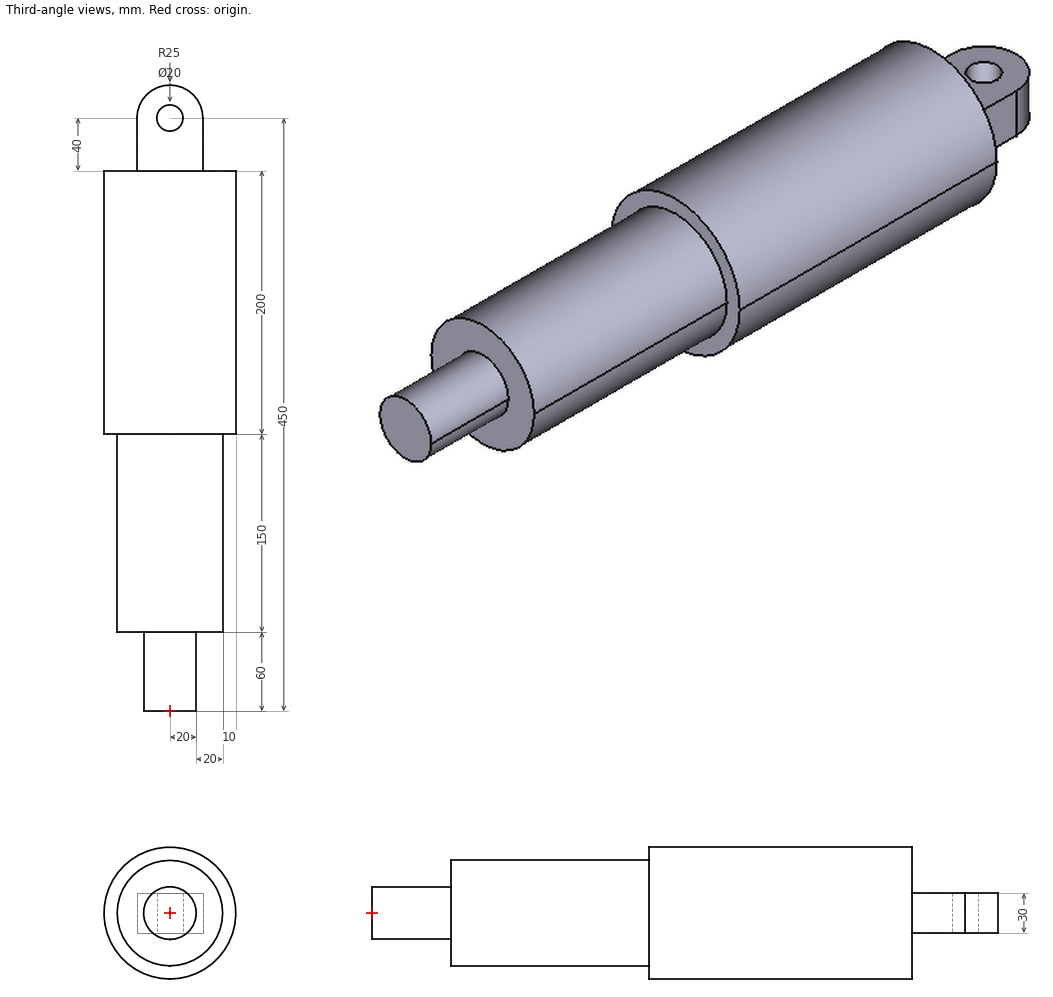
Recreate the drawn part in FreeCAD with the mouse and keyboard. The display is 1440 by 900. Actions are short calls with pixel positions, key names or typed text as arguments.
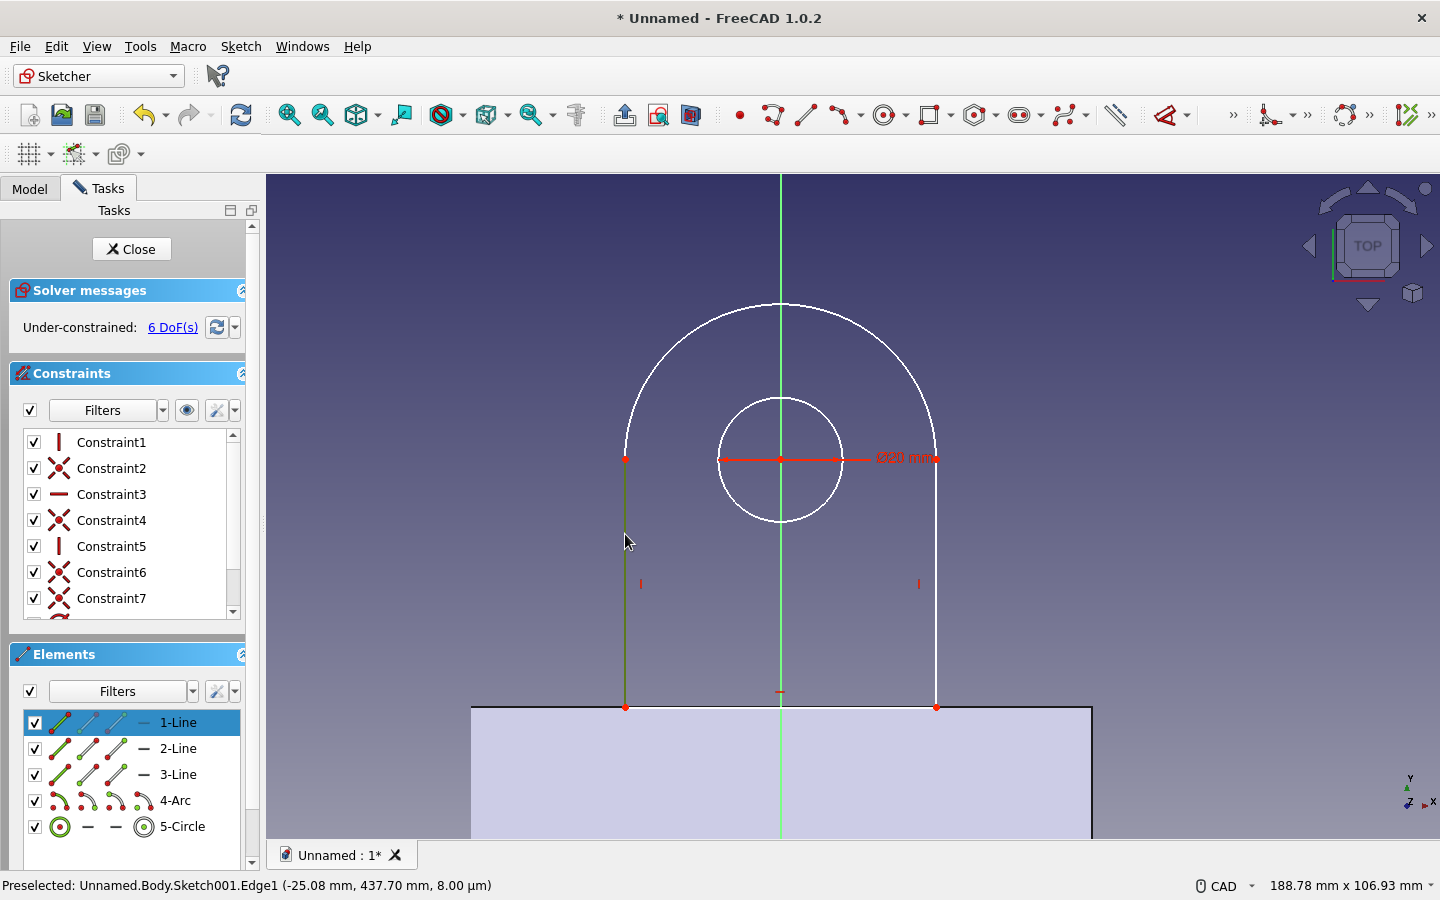
click(872, 334)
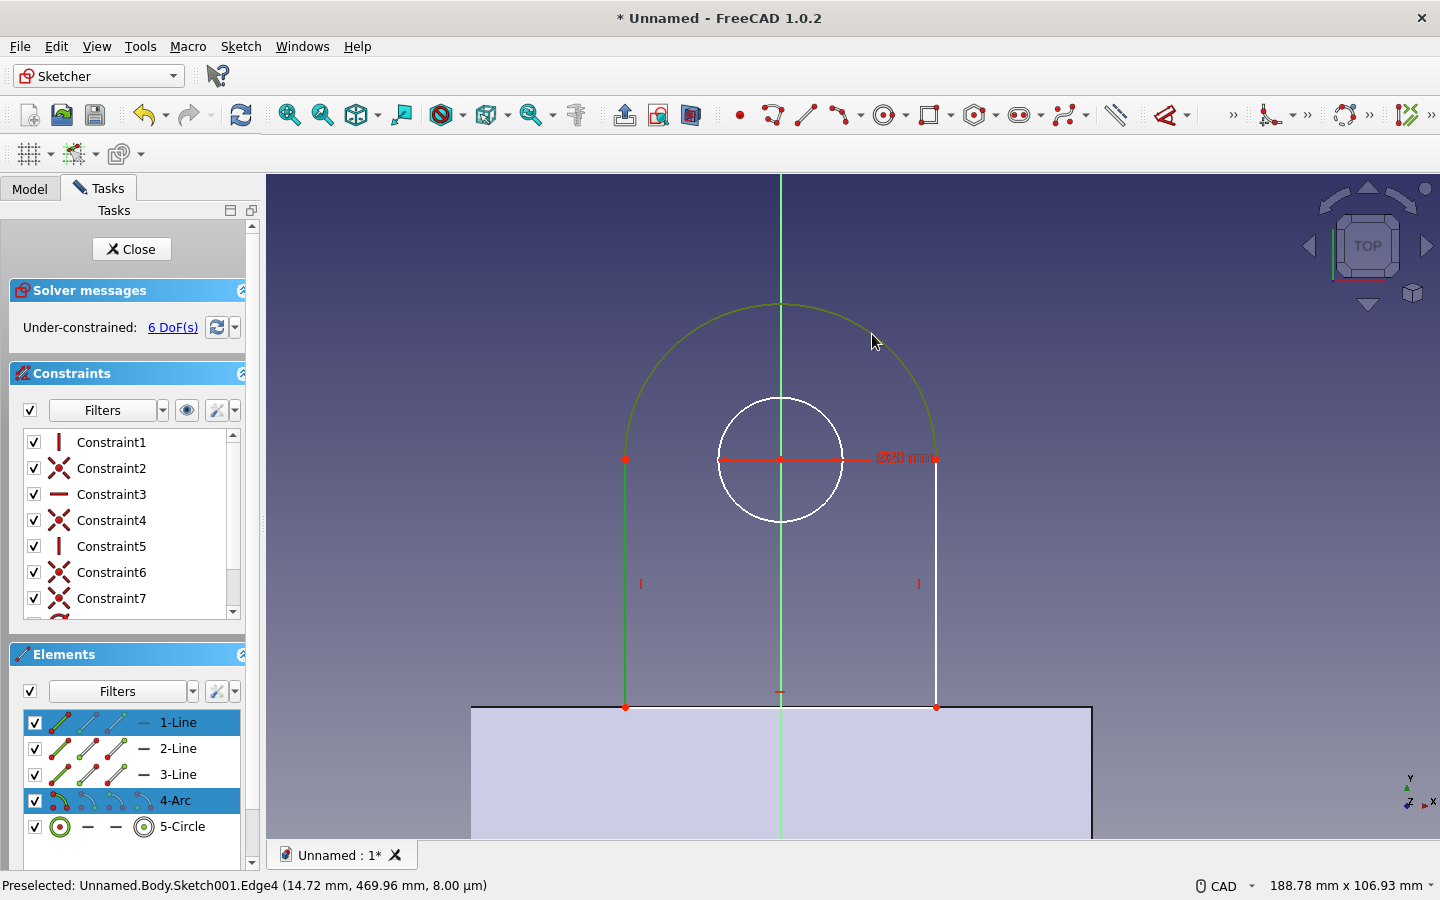
key(t)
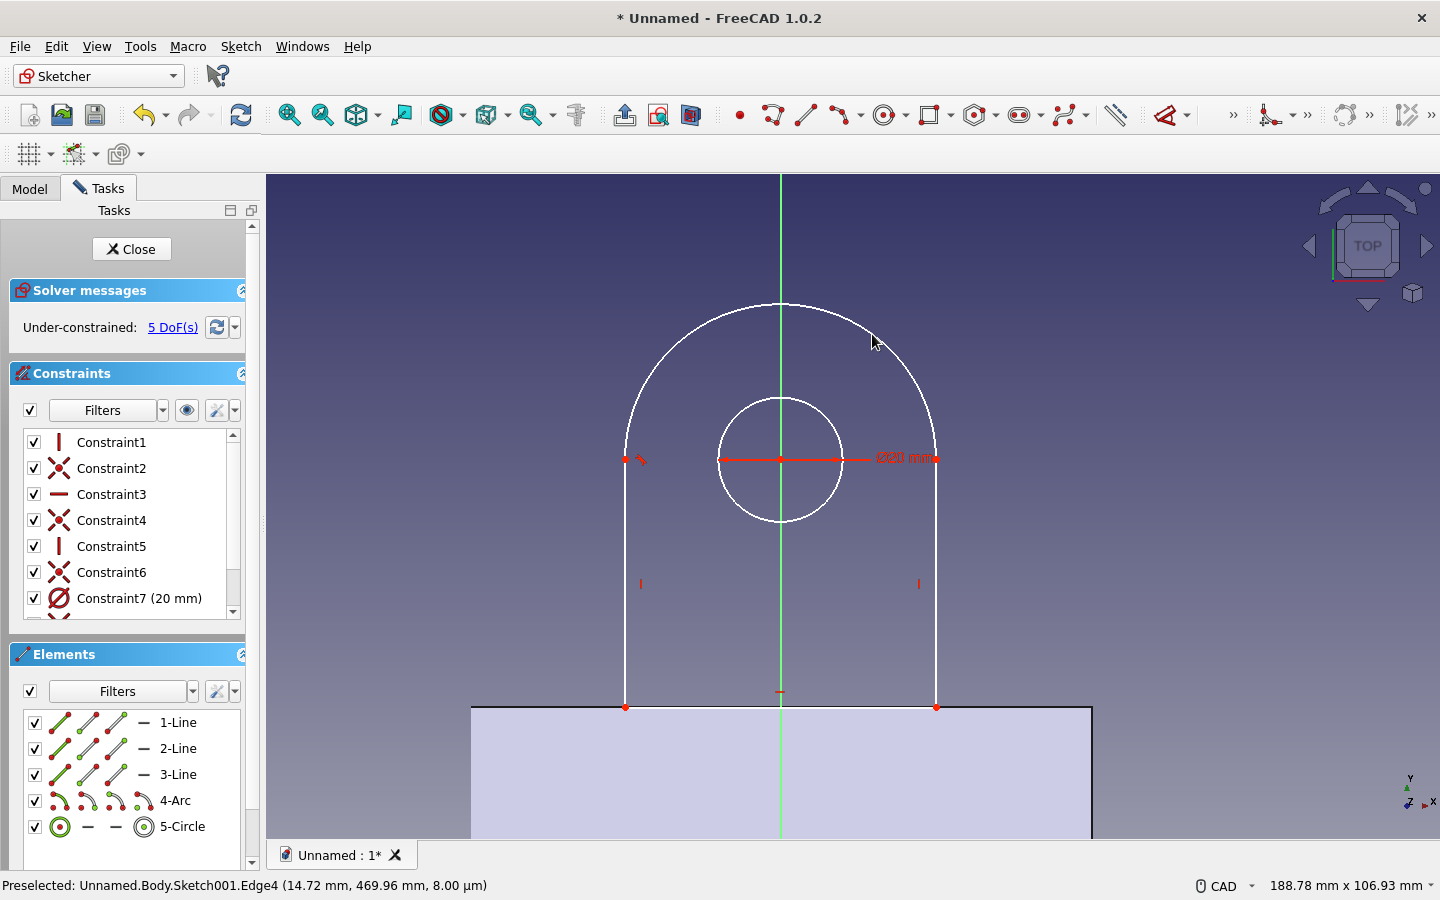
click(936, 634)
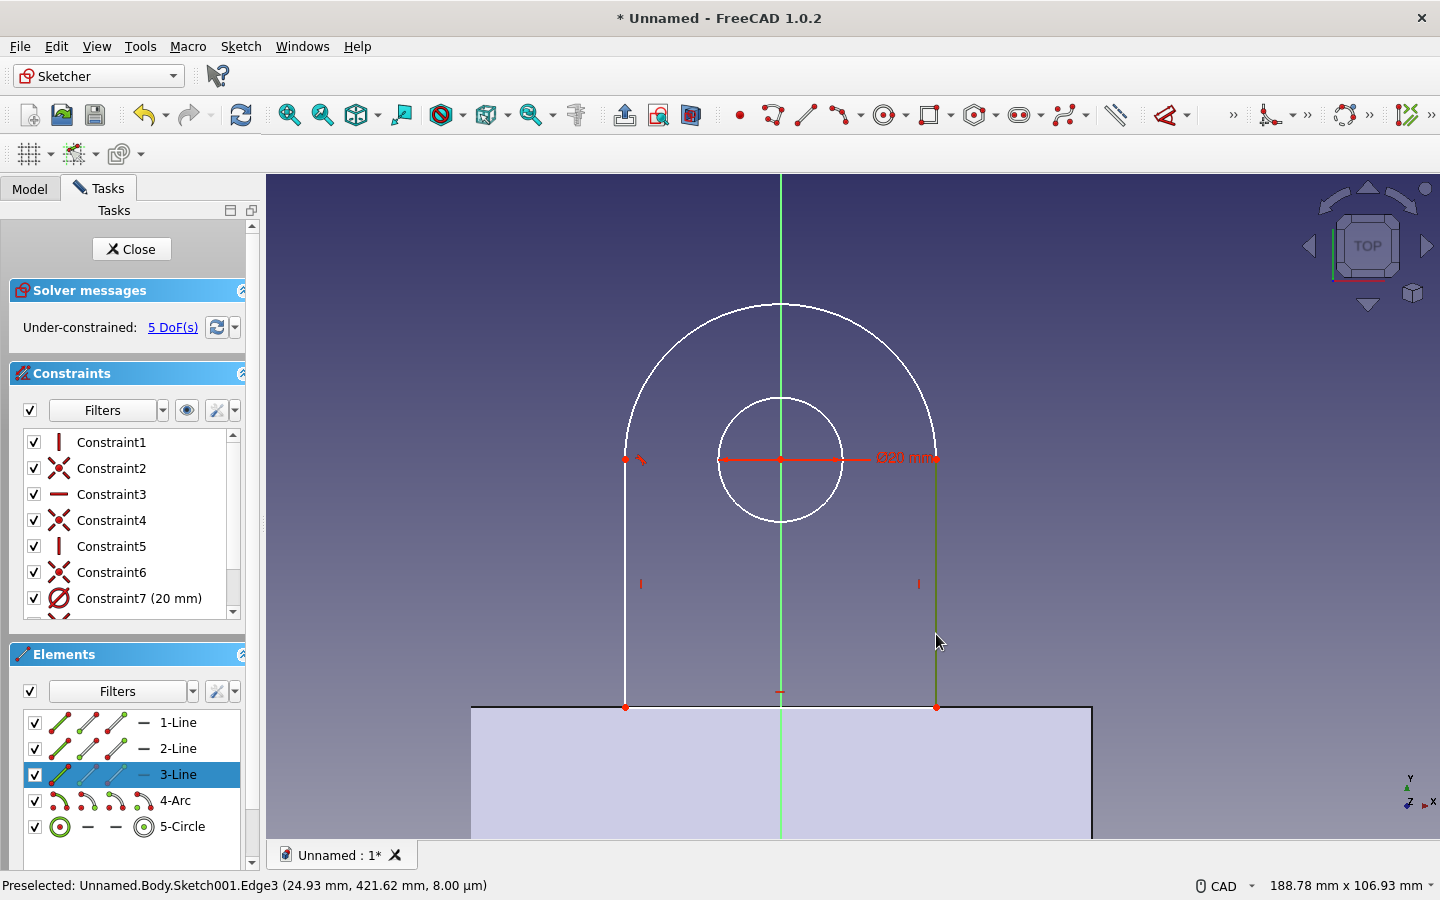
click(872, 334)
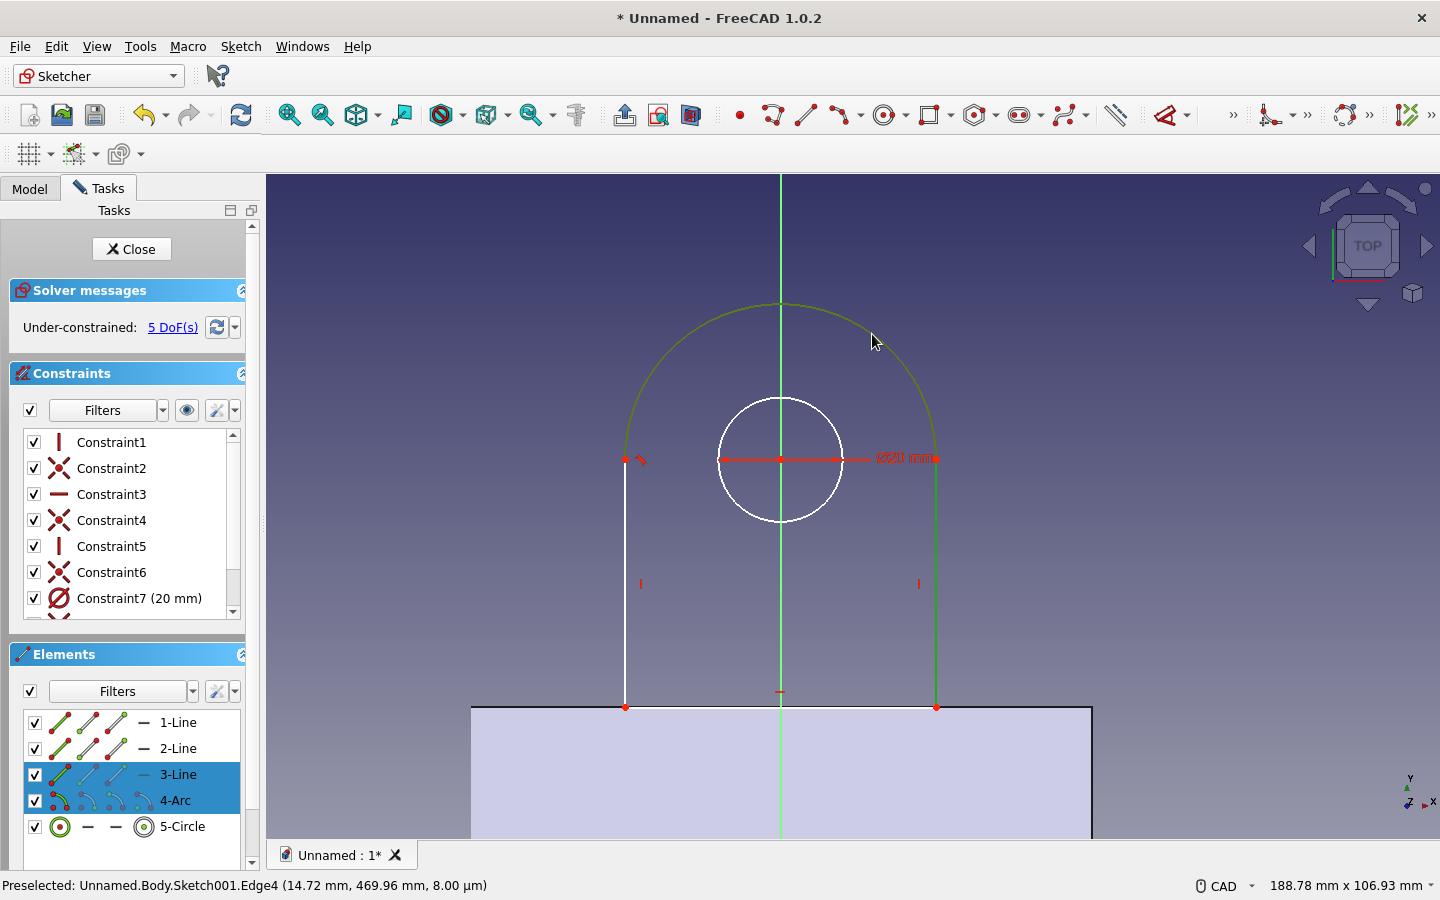
key(t)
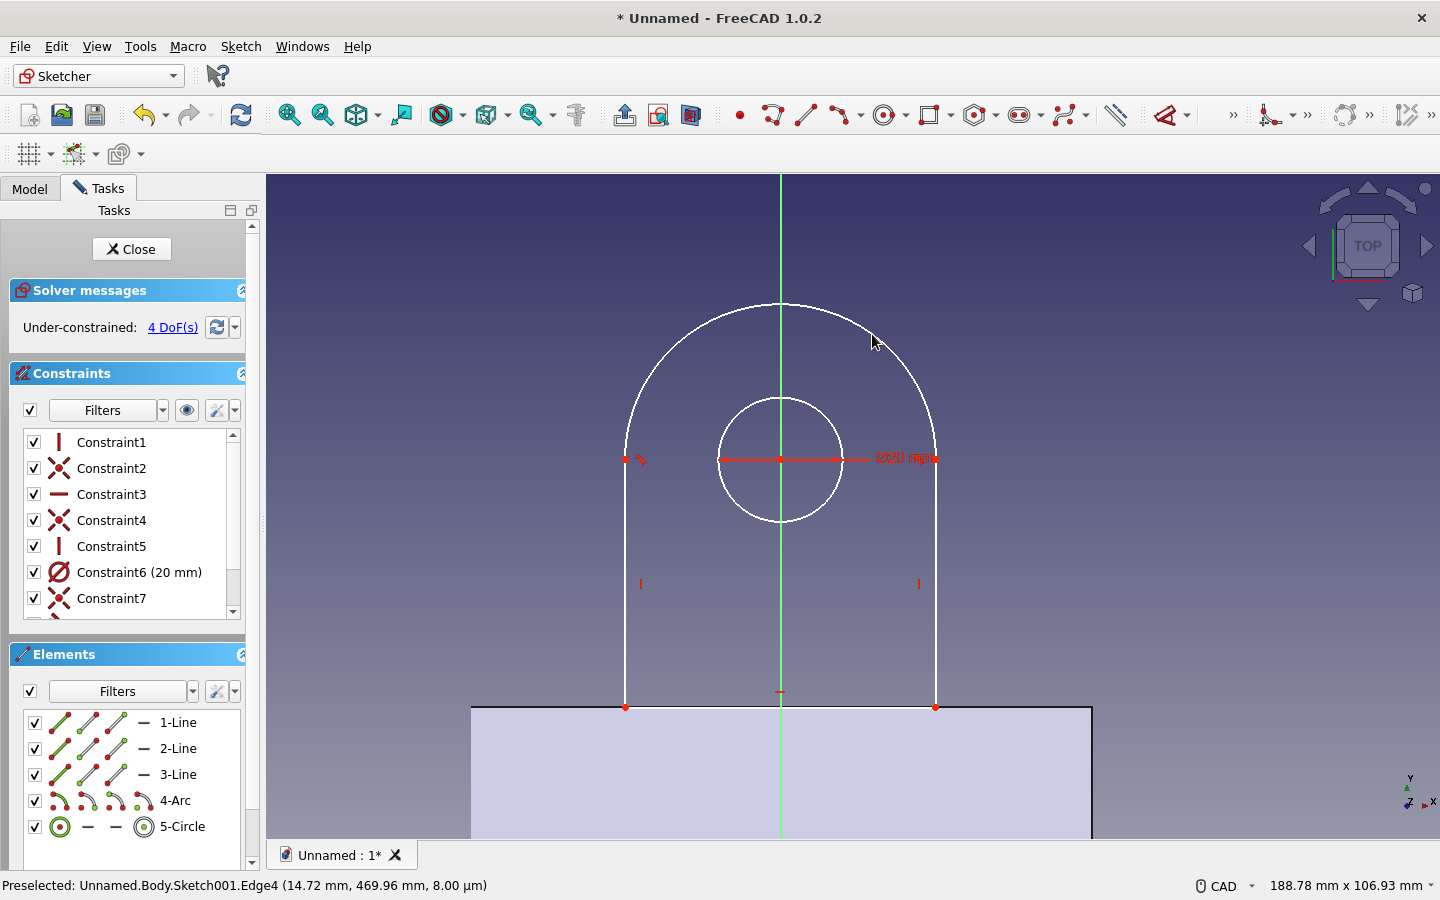
click(780, 460)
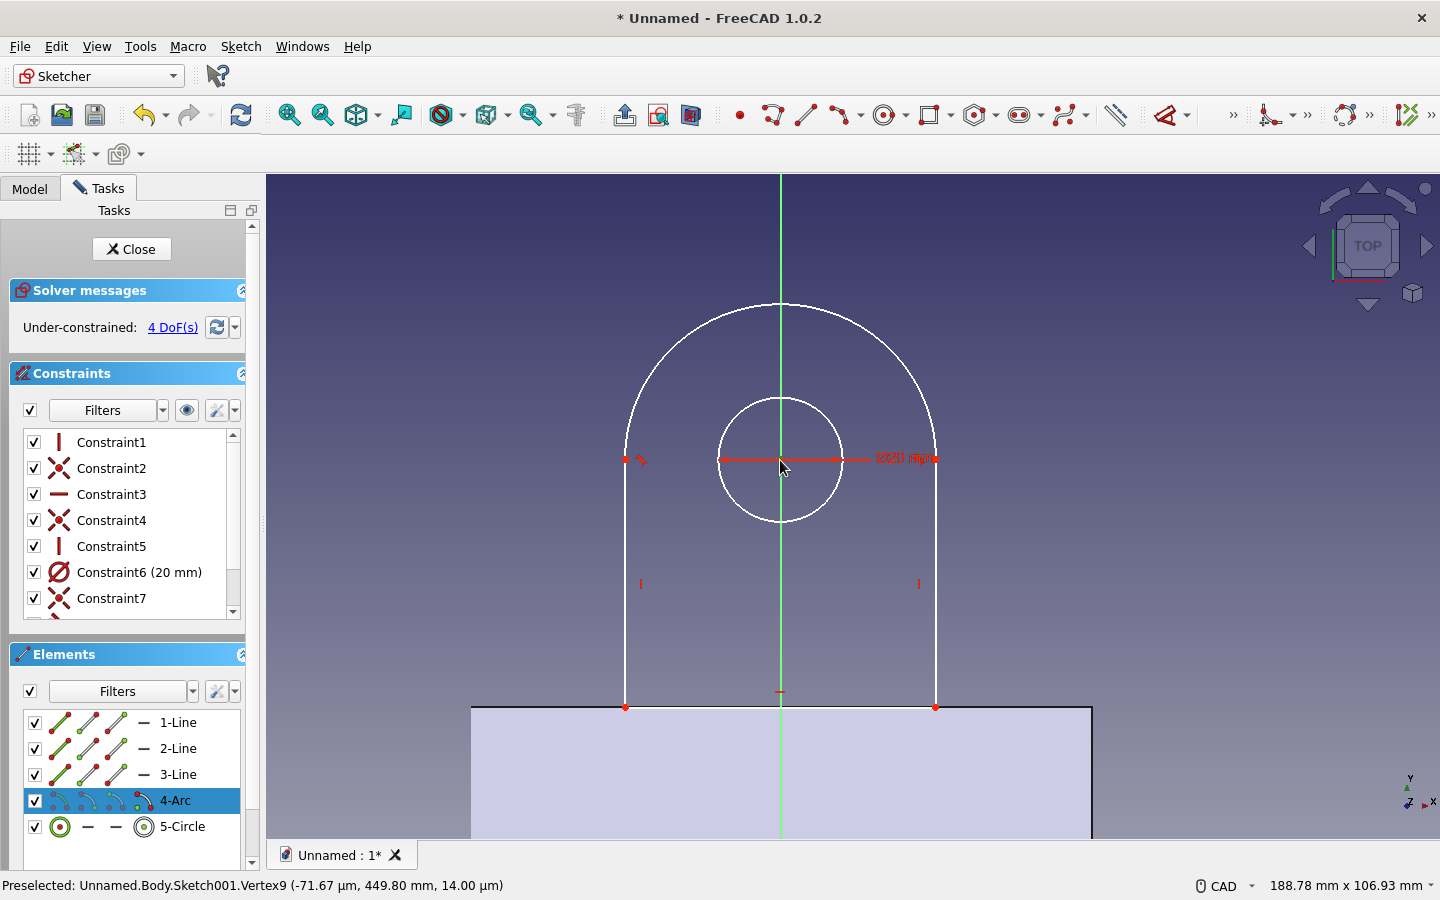
click(781, 767)